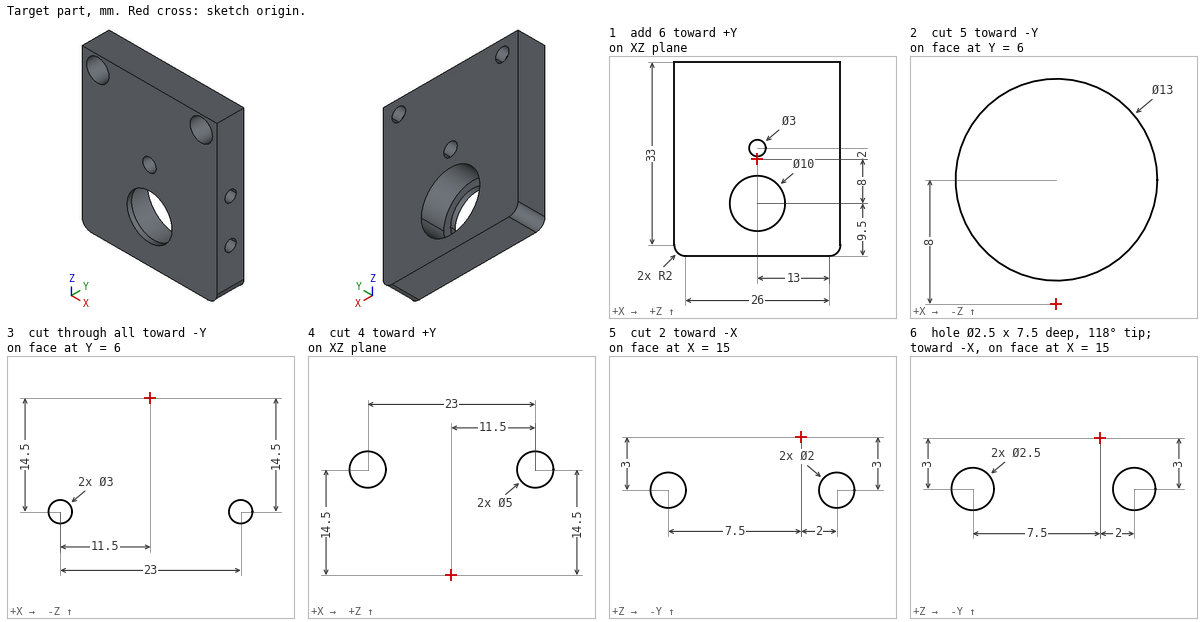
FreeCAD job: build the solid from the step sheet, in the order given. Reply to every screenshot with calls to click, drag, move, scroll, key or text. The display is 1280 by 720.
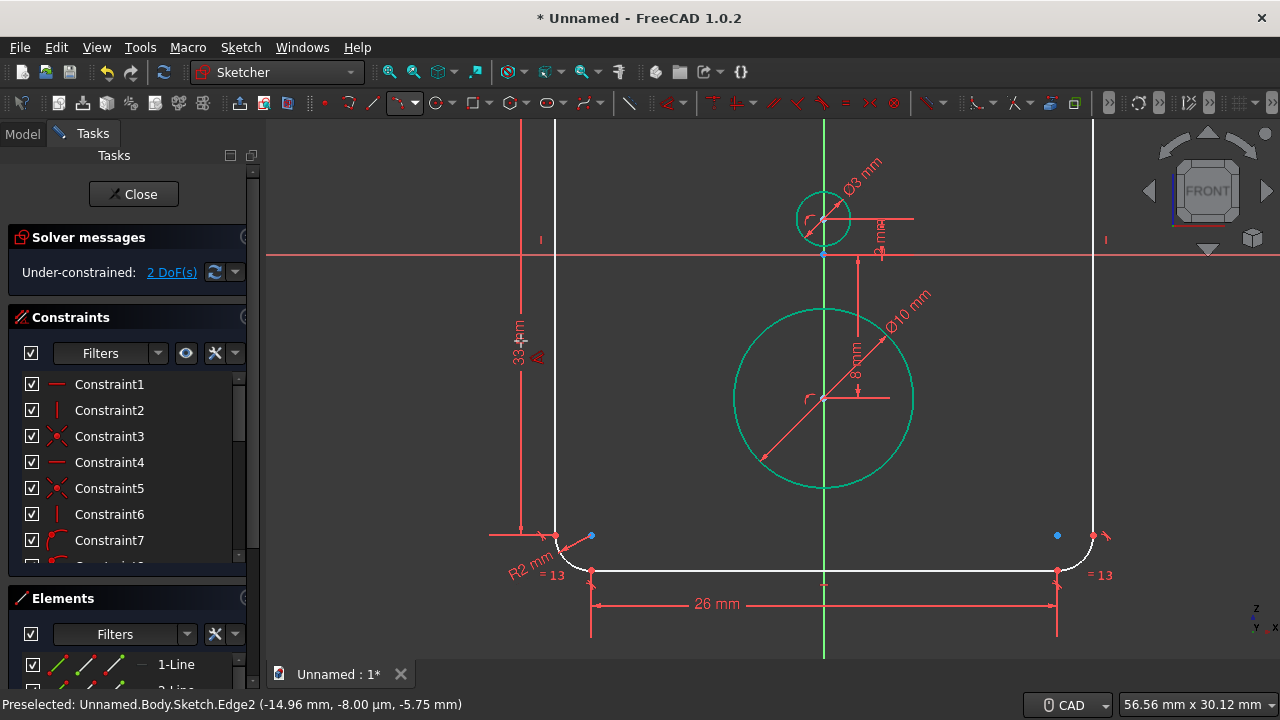
click(1057, 571)
click(941, 605)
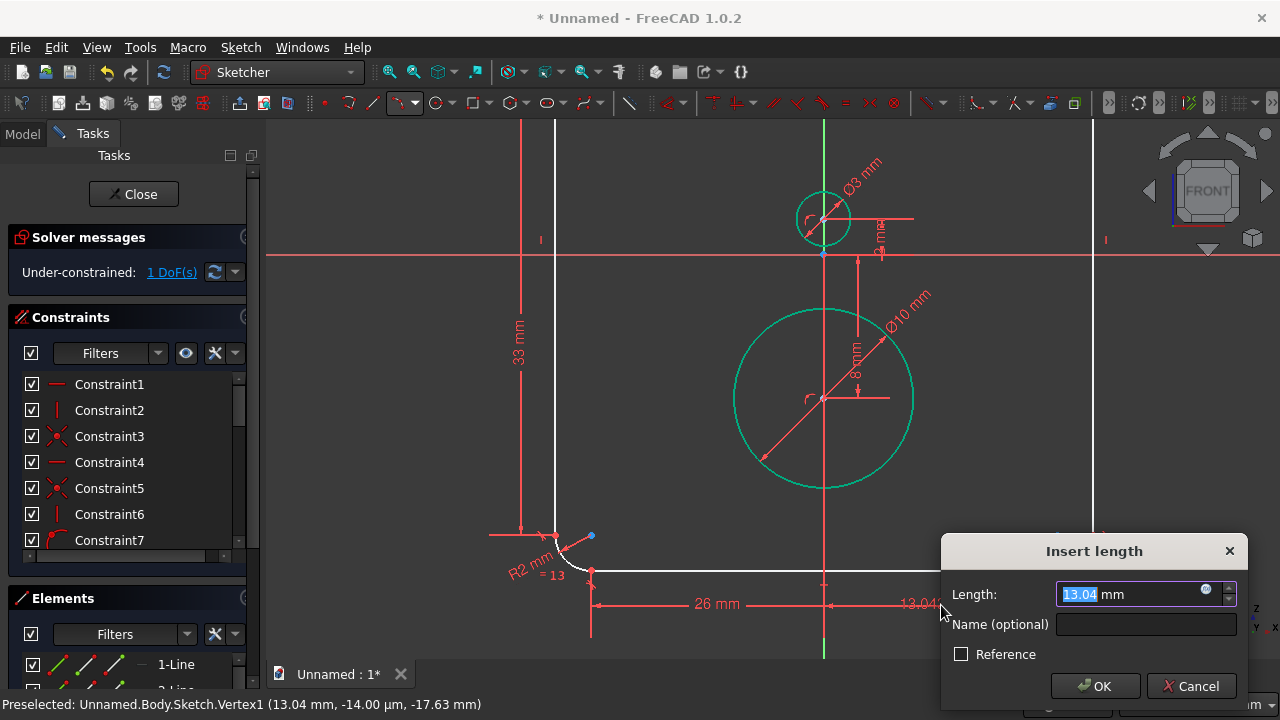
text(13)
key(Return)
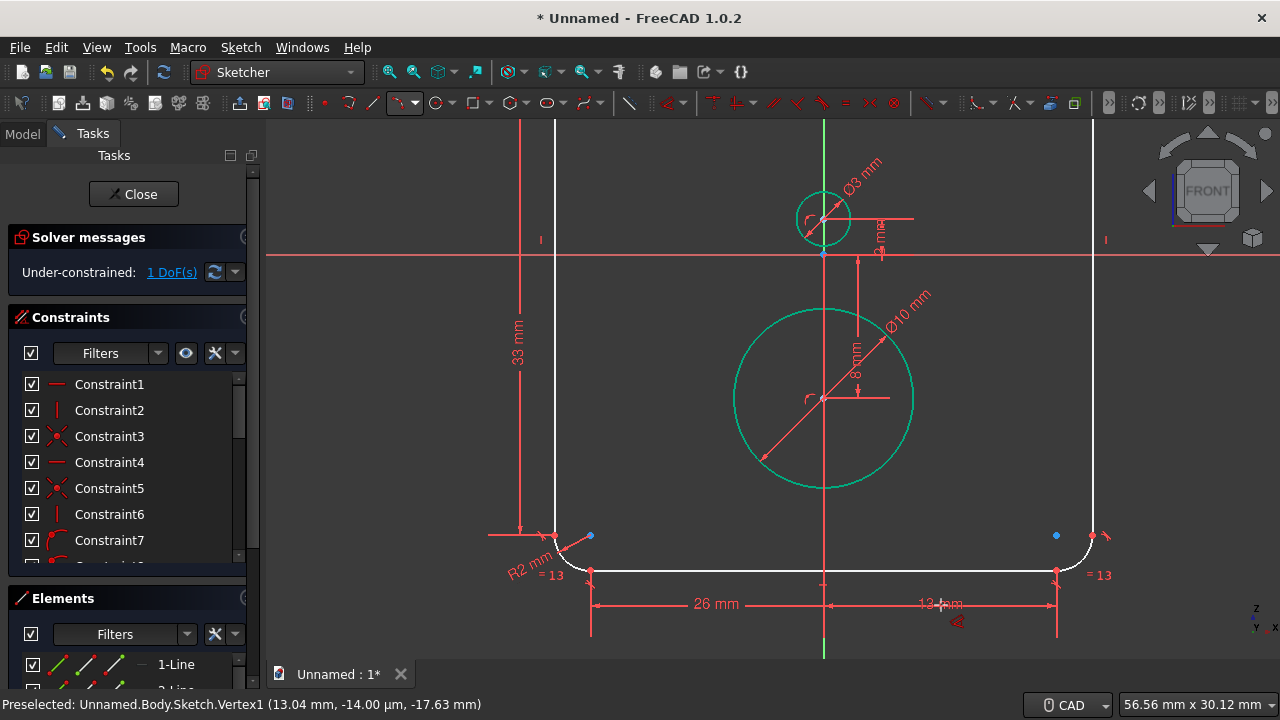
click(1057, 571)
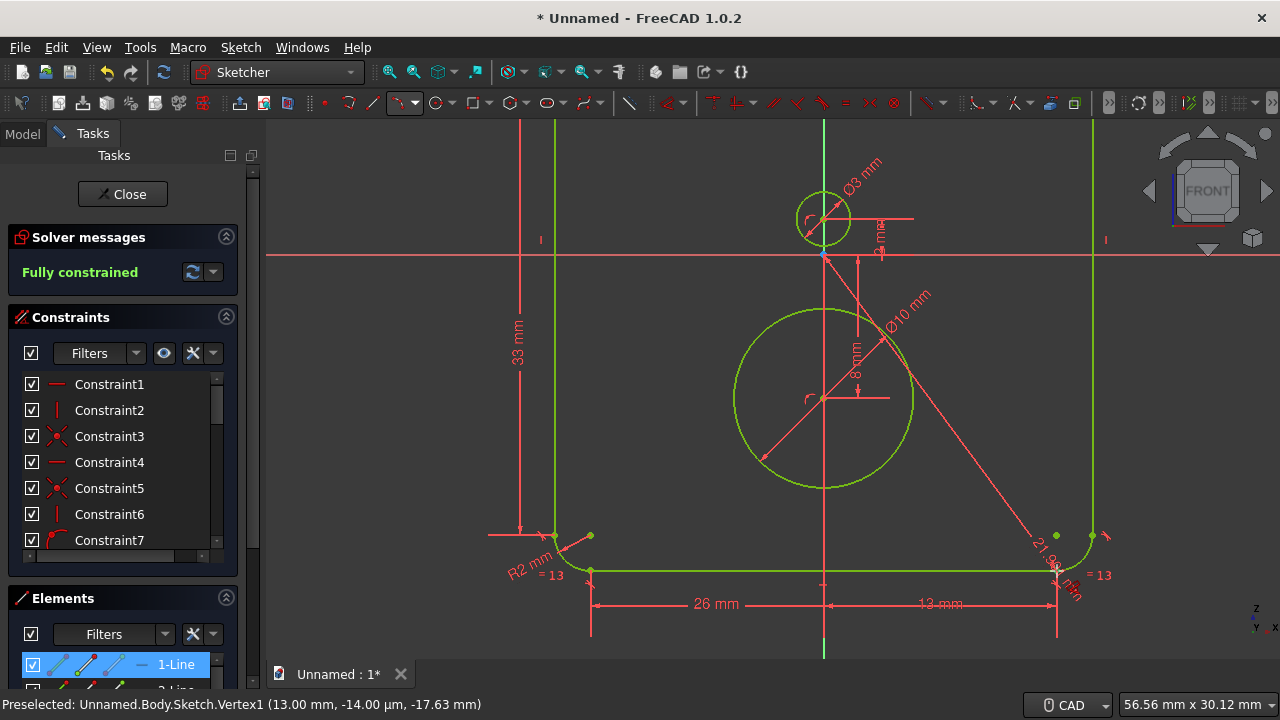
click(824, 398)
click(790, 445)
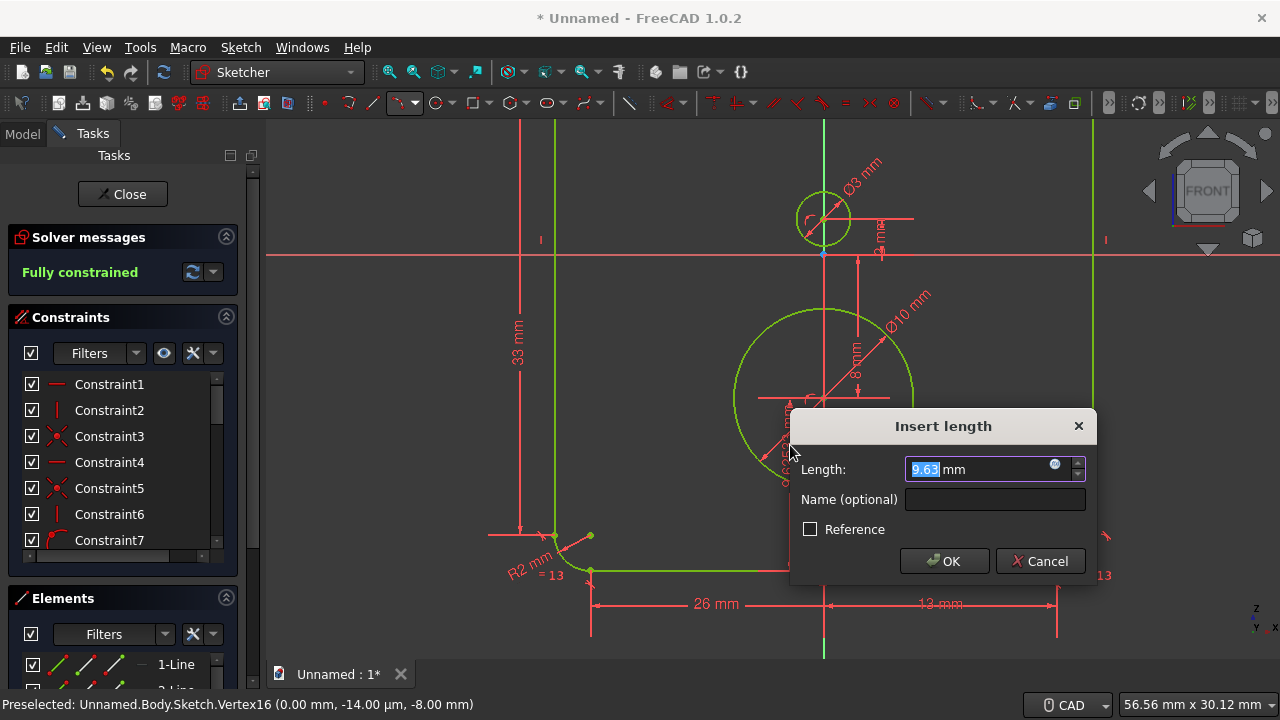
text(9.5)
key(Return)
key(Escape)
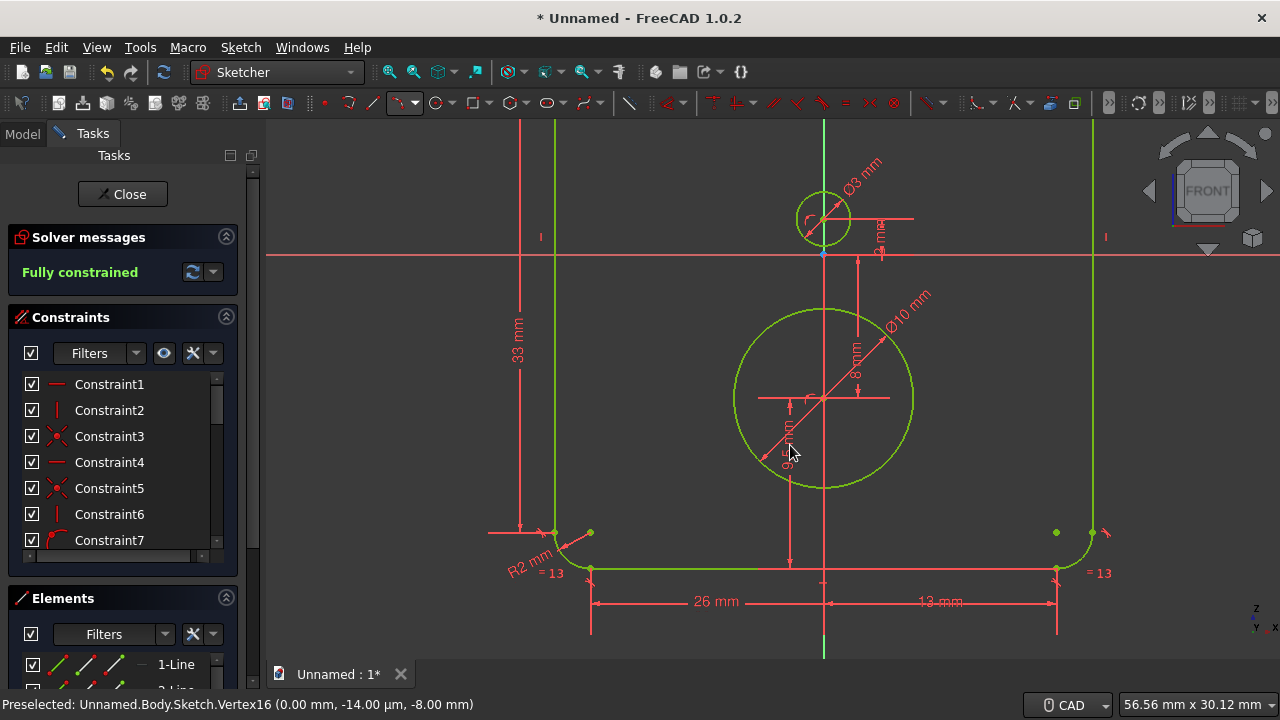
click(123, 194)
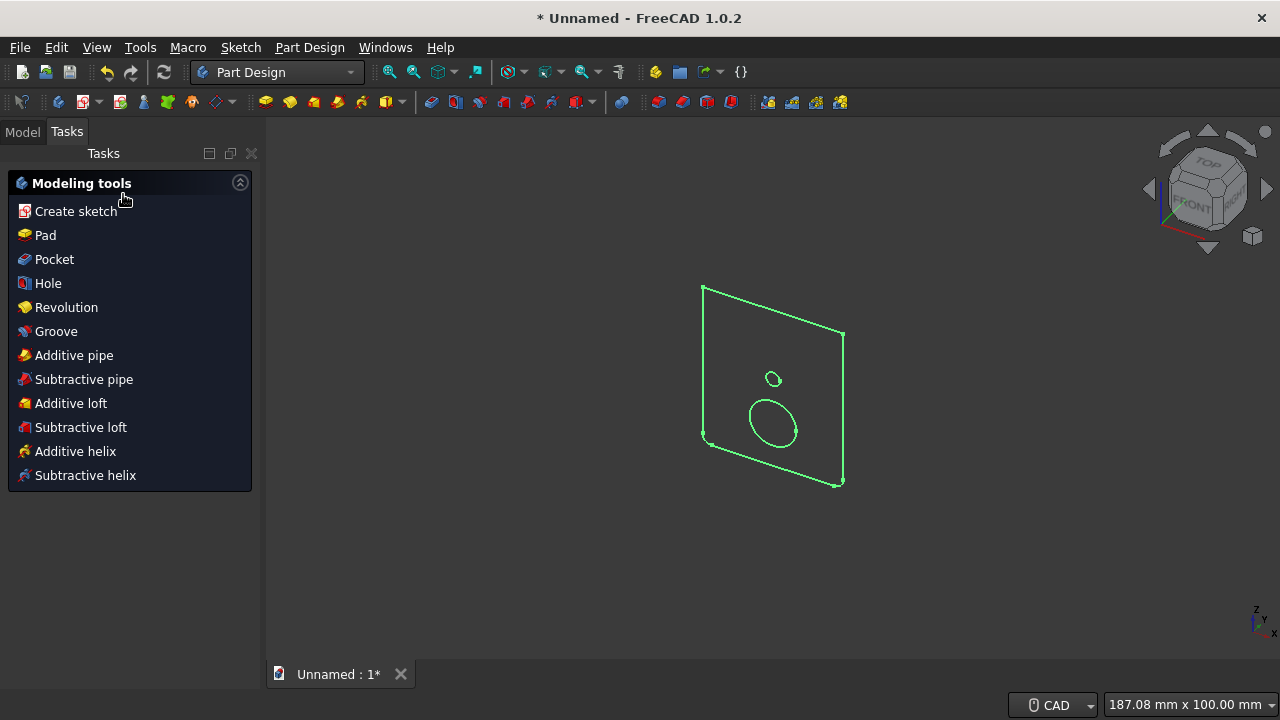
click(266, 102)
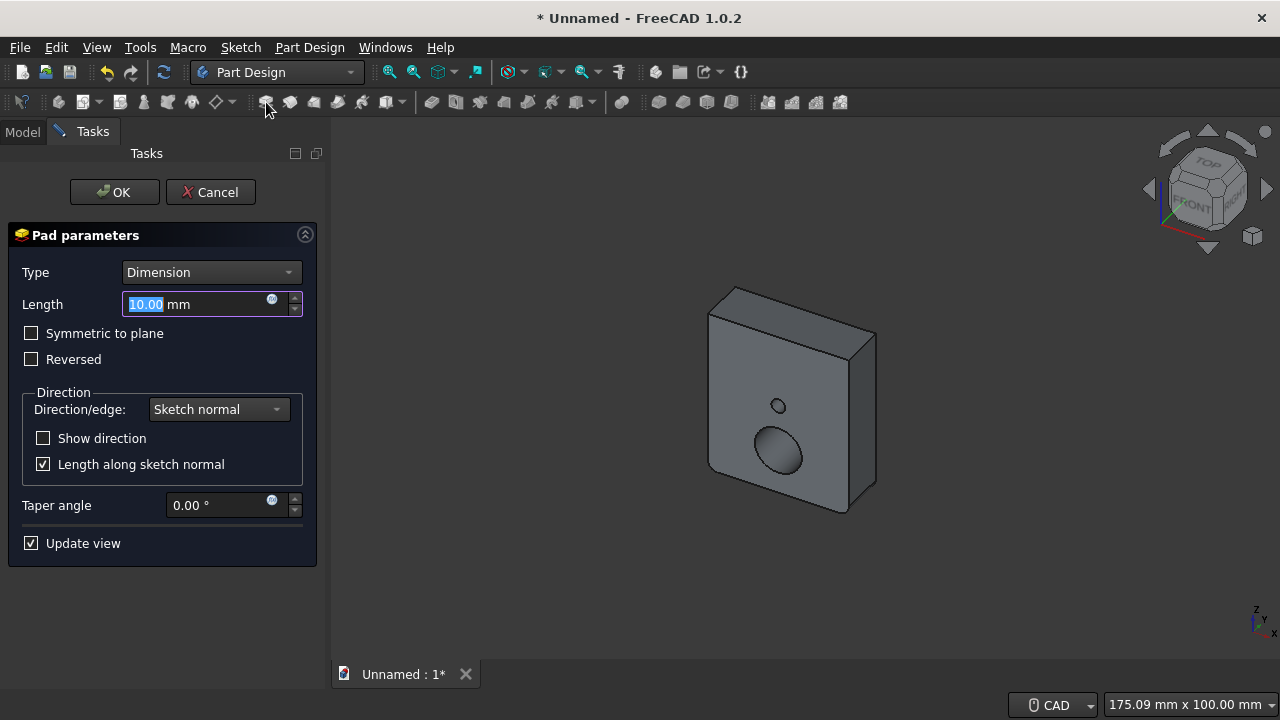
text(6)
key(Tab)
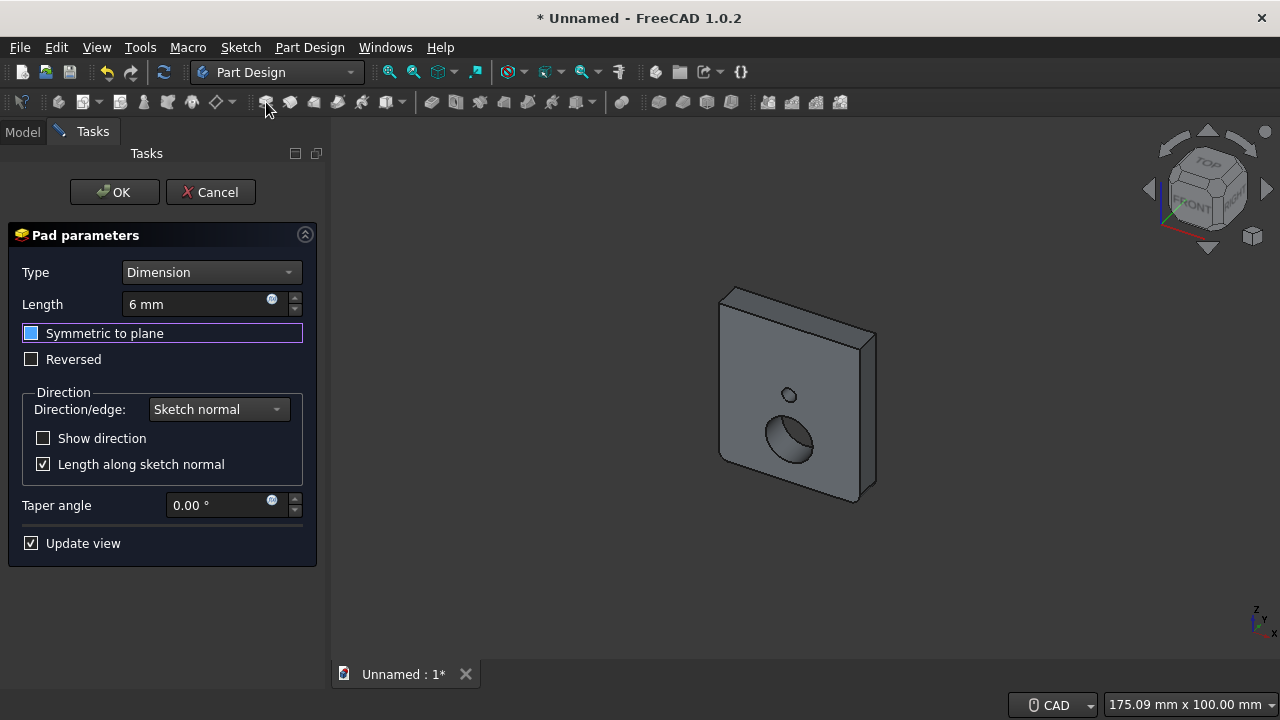
click(30, 359)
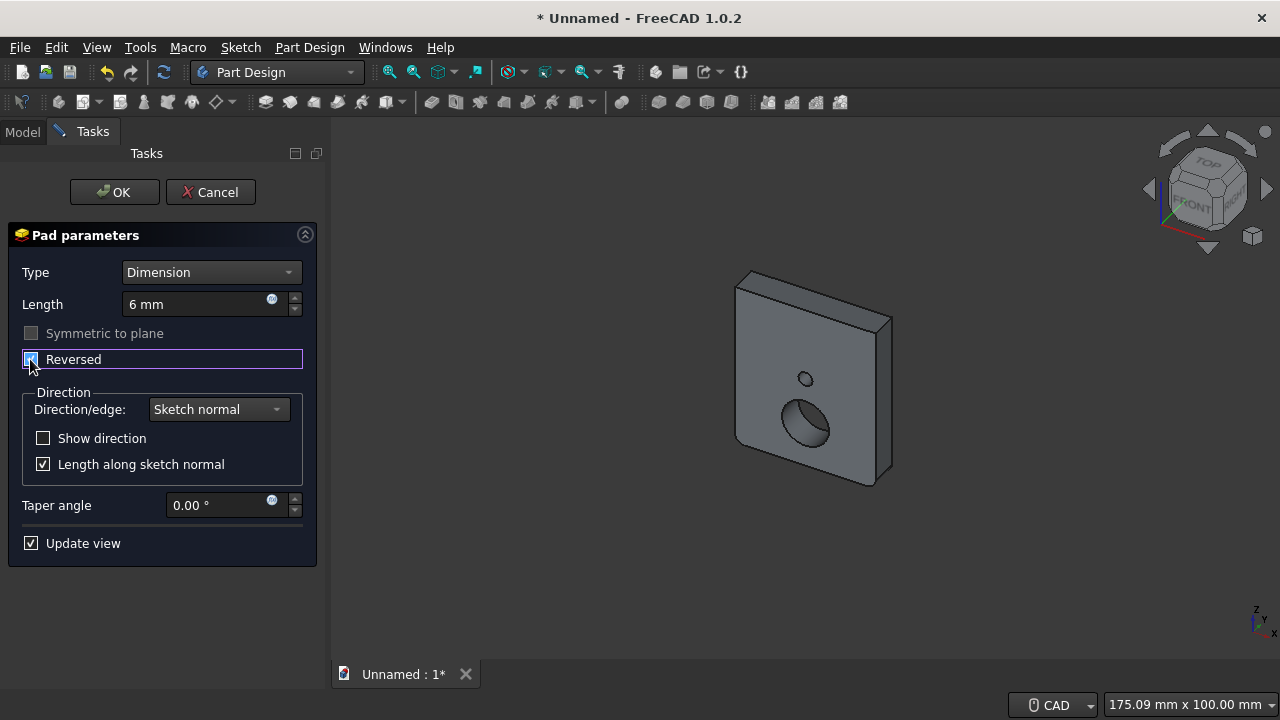
click(115, 192)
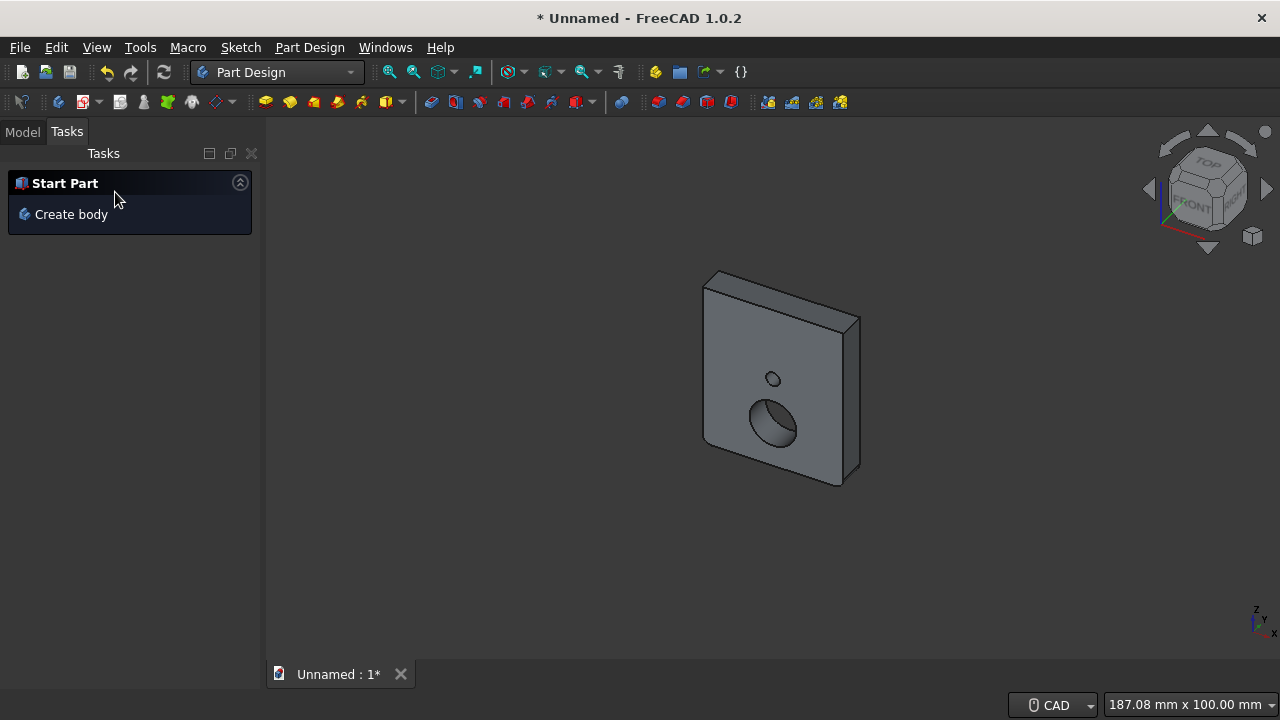
key(v)
key(f)